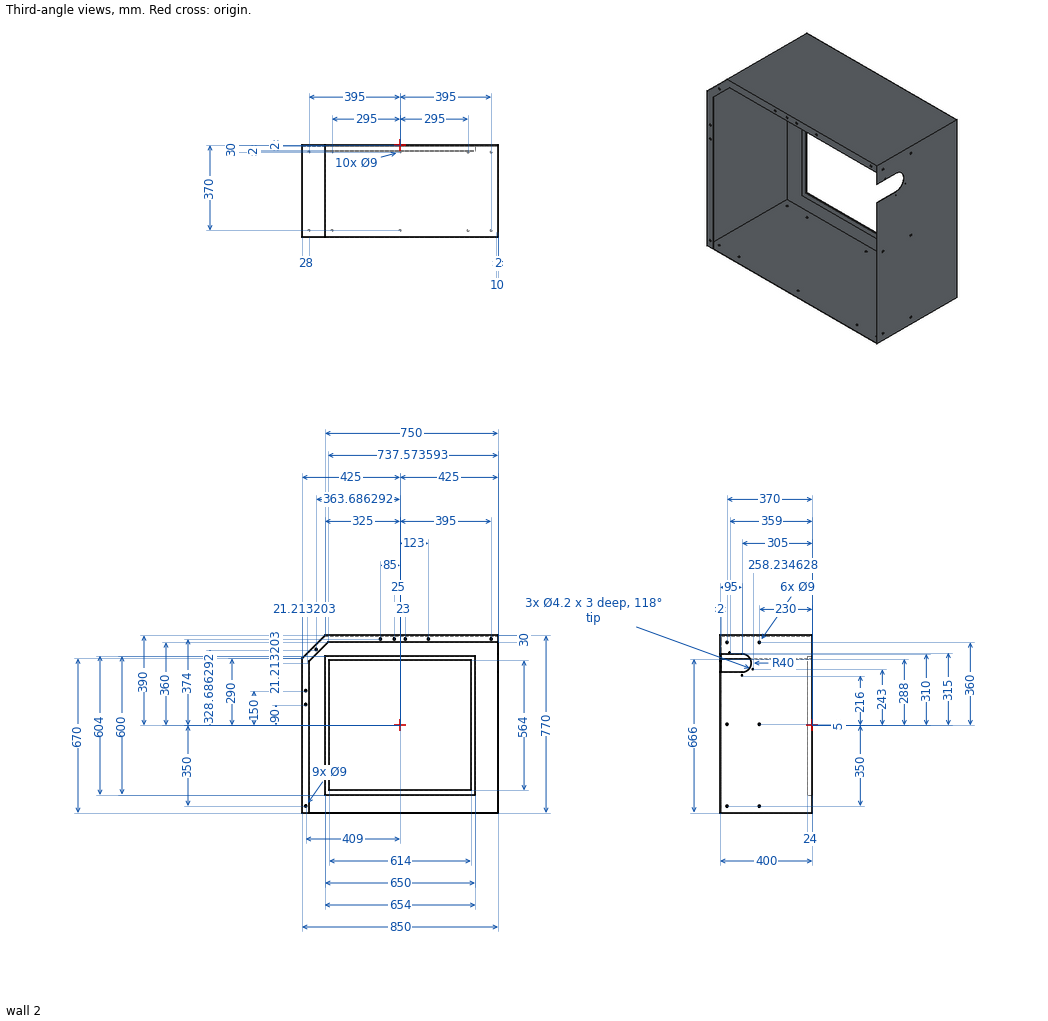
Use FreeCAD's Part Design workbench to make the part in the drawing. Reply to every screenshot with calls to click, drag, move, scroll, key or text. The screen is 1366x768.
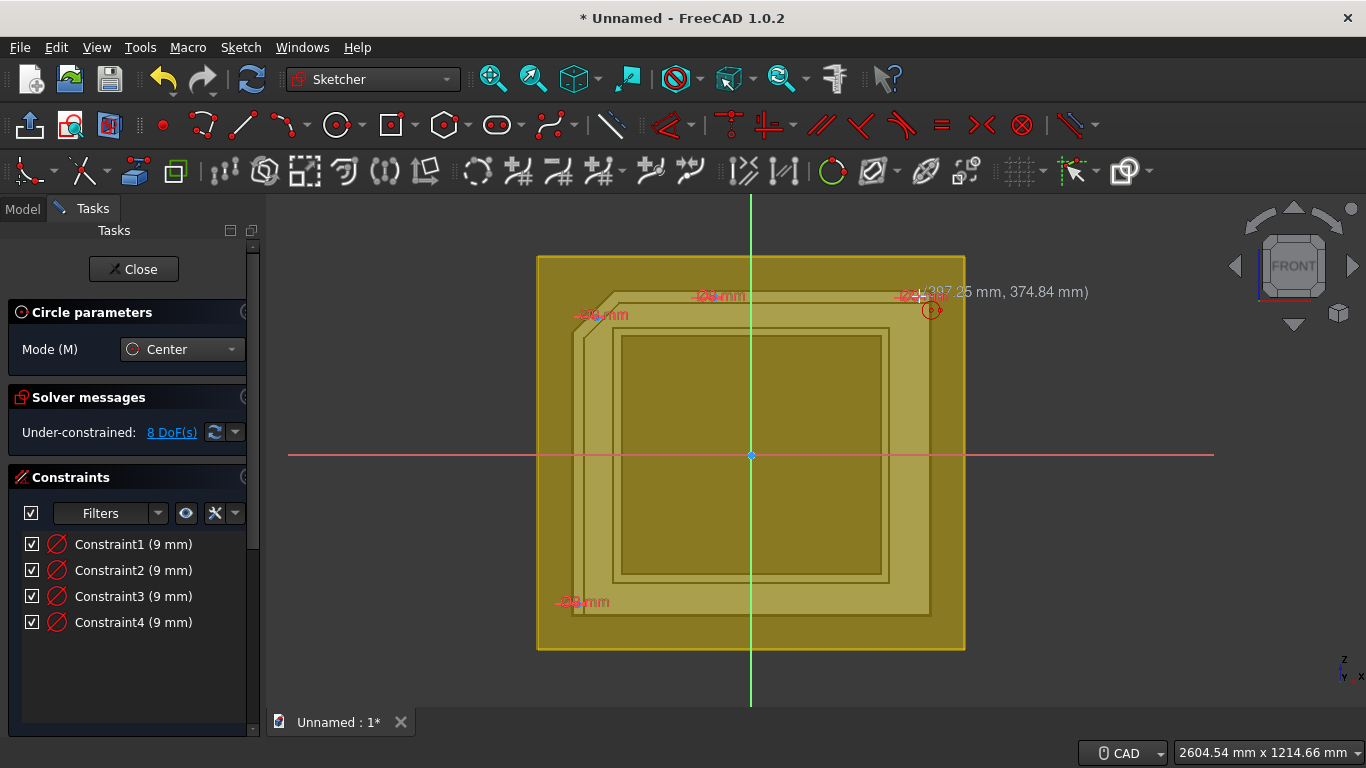
scroll(578, 417, up, 13)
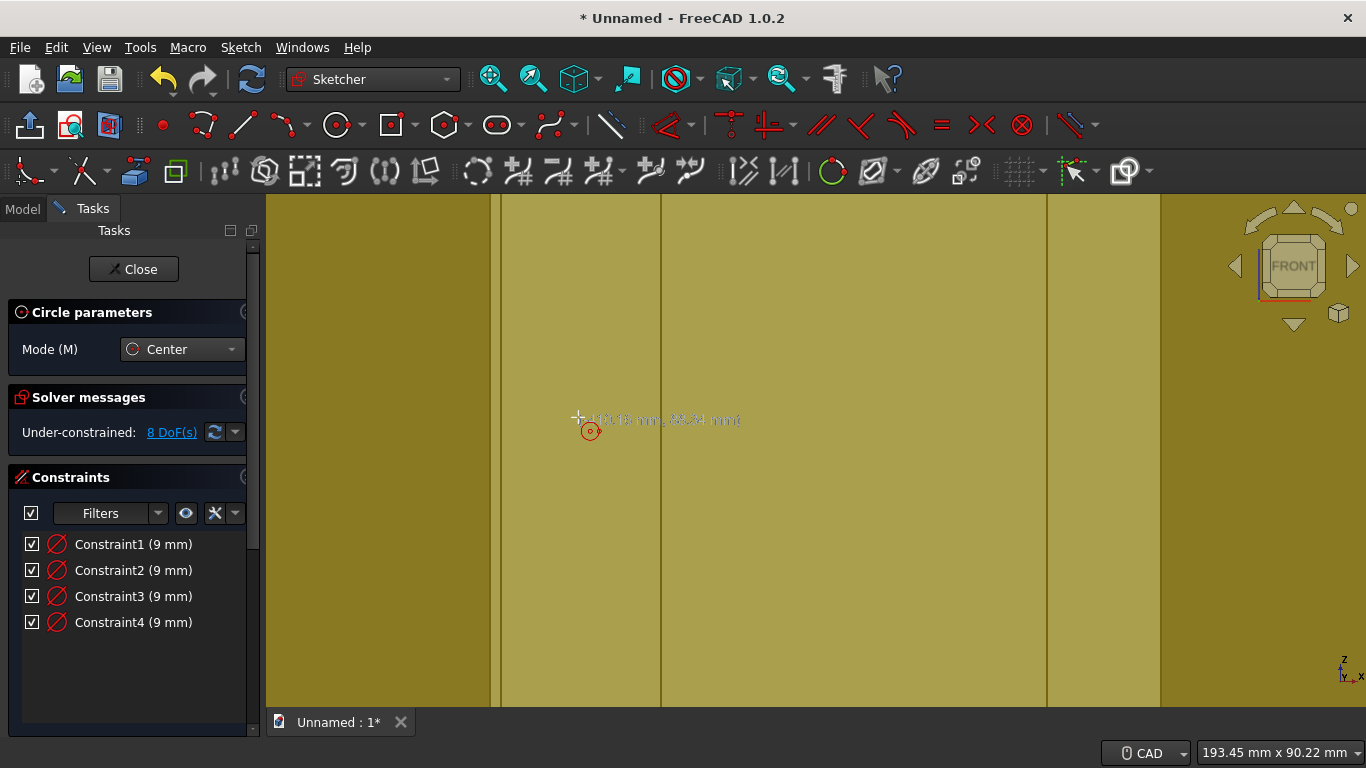
scroll(577, 418, down, 13)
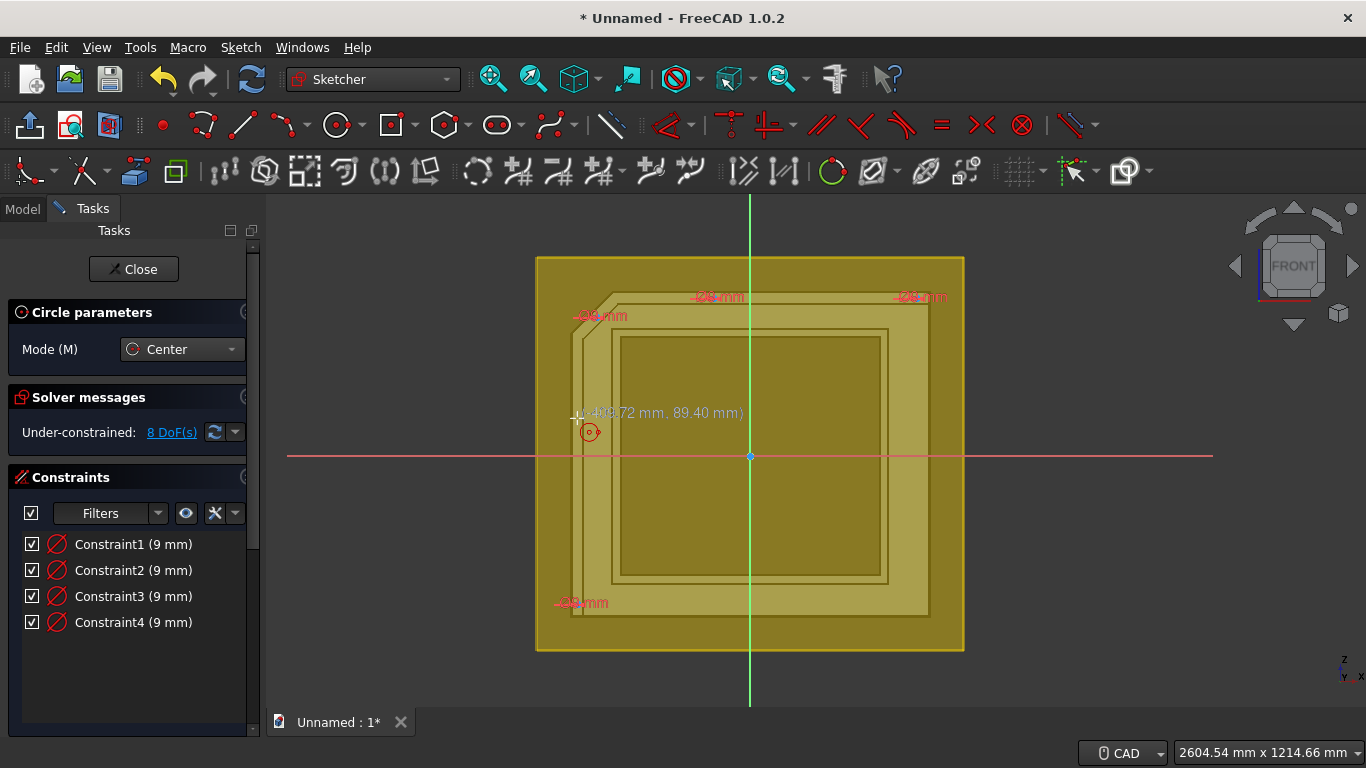
click(578, 418)
move(579, 417)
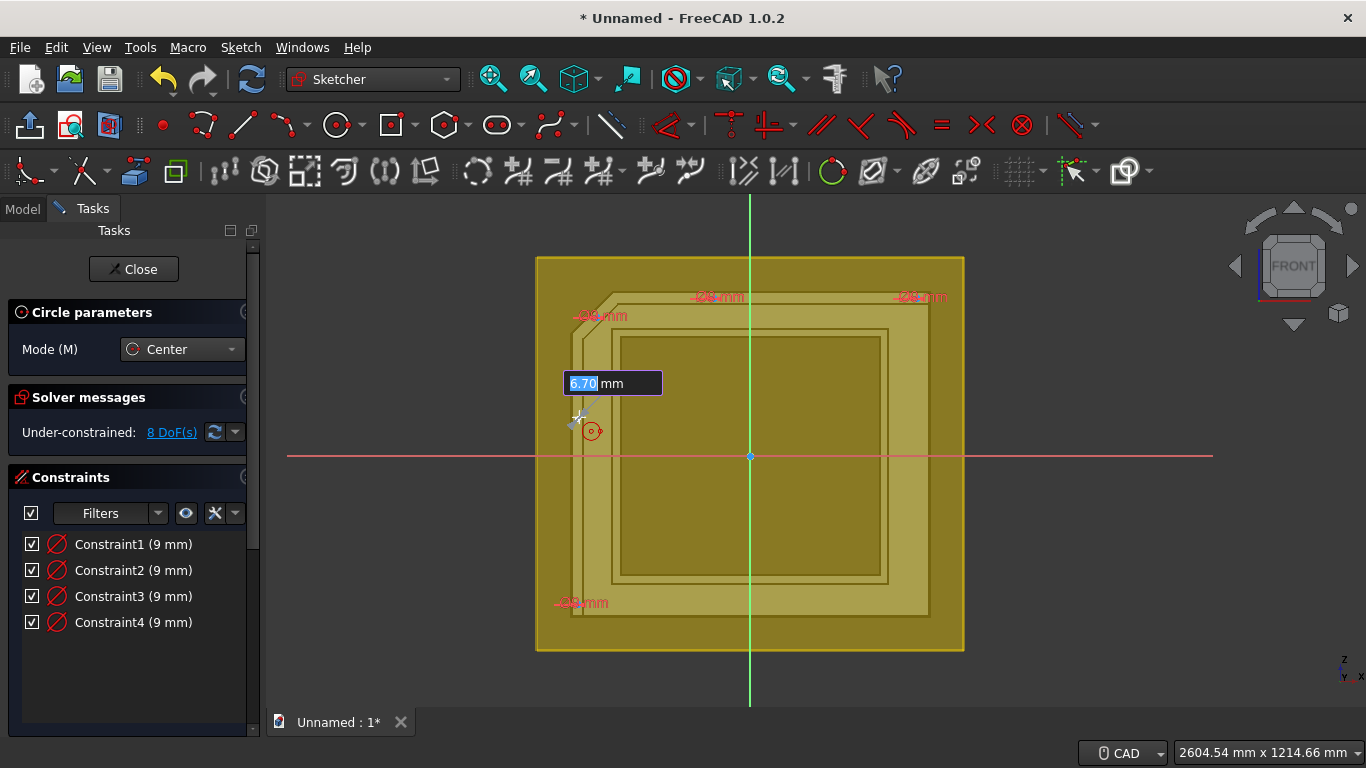
text(9)
key(Return)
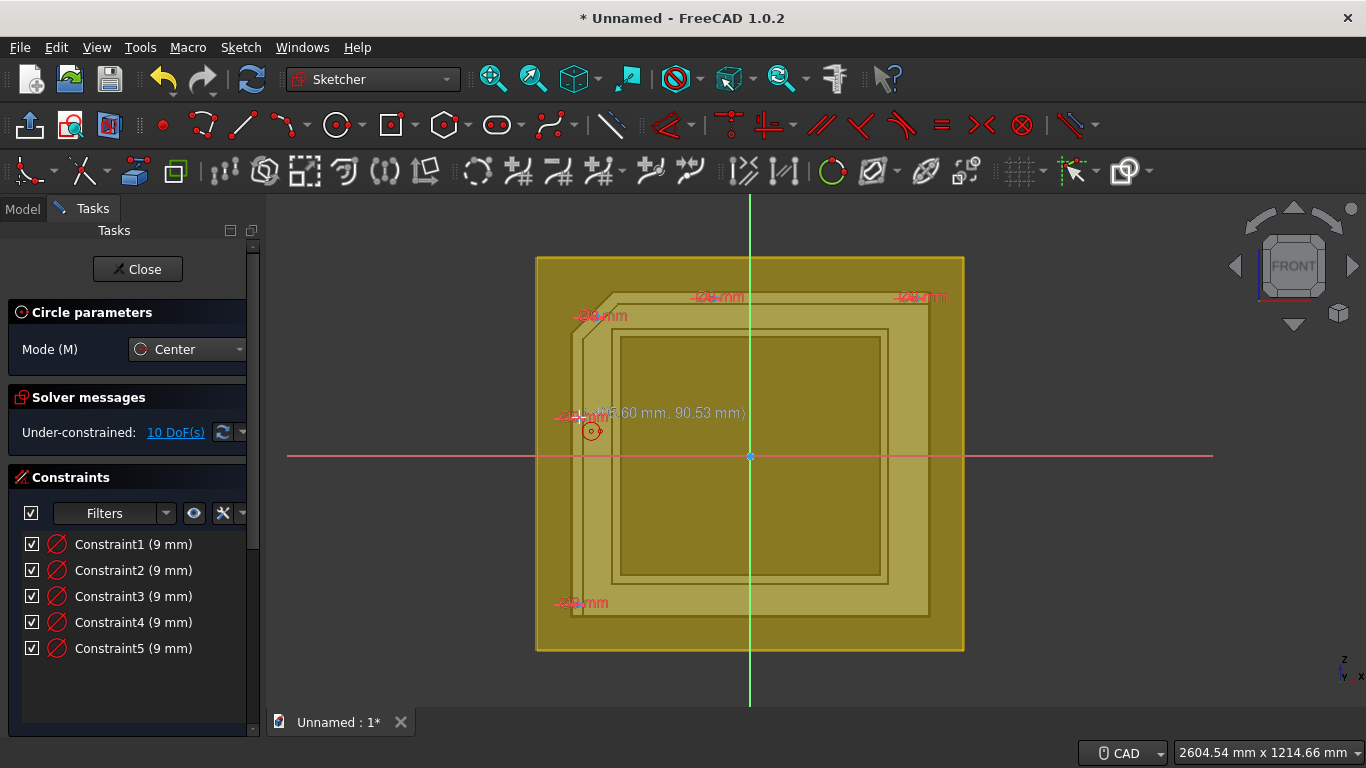
scroll(740, 298, up, 13)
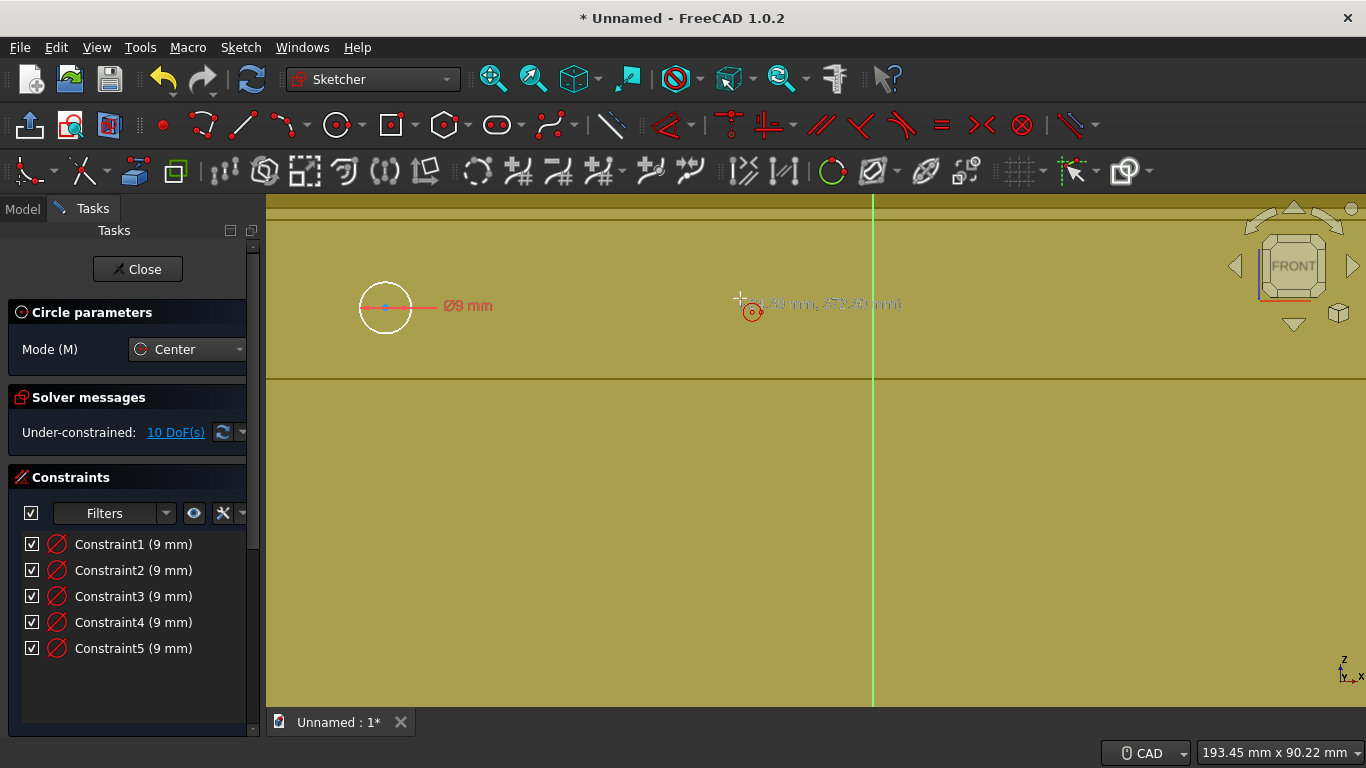
scroll(741, 297, down, 13)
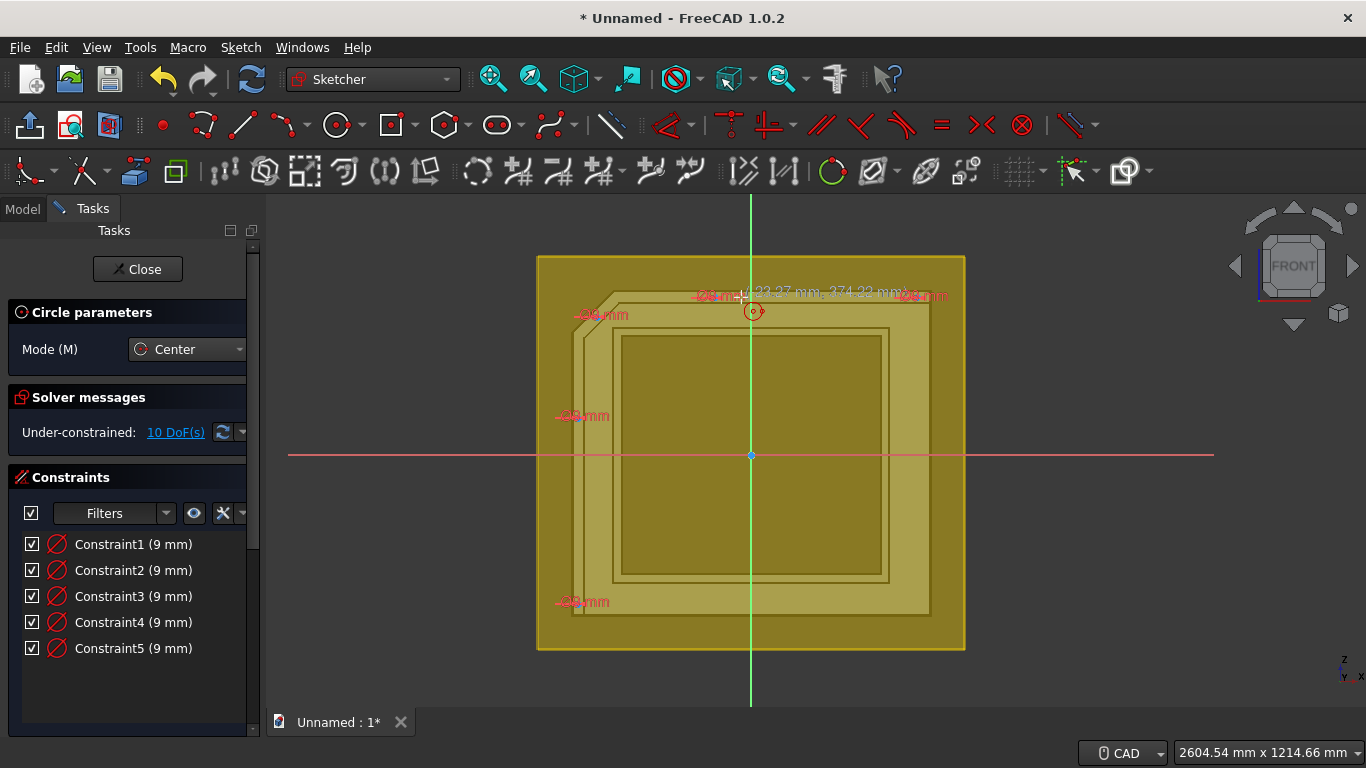
scroll(741, 297, up, 3)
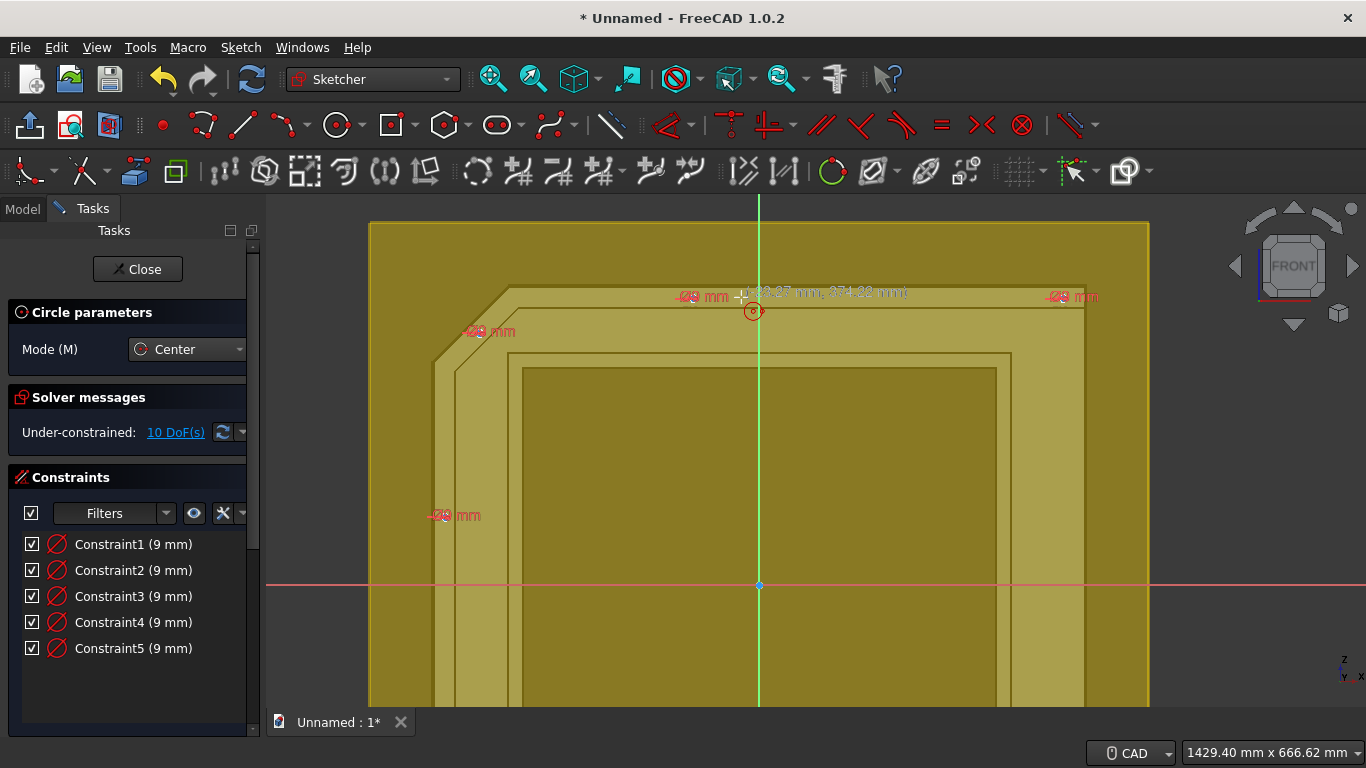
click(740, 297)
move(742, 295)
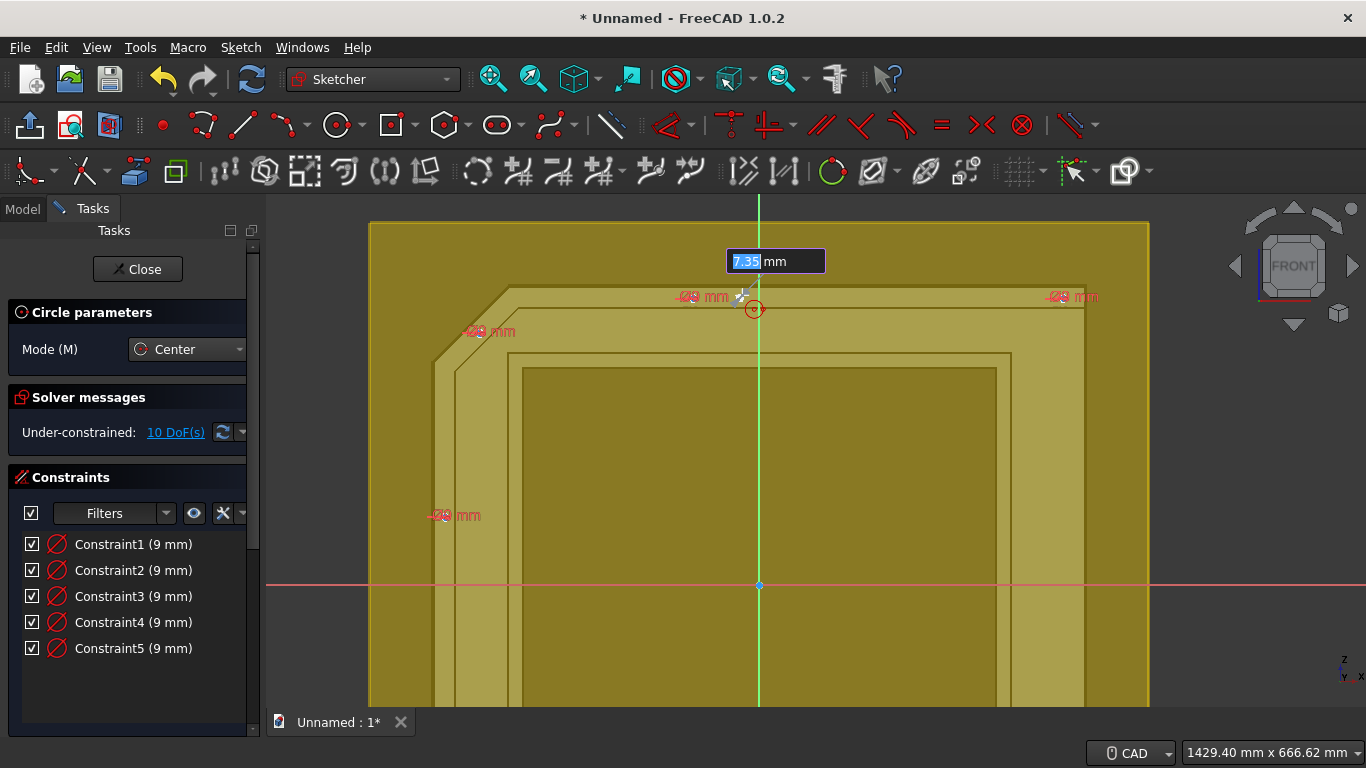
text(9)
key(Return)